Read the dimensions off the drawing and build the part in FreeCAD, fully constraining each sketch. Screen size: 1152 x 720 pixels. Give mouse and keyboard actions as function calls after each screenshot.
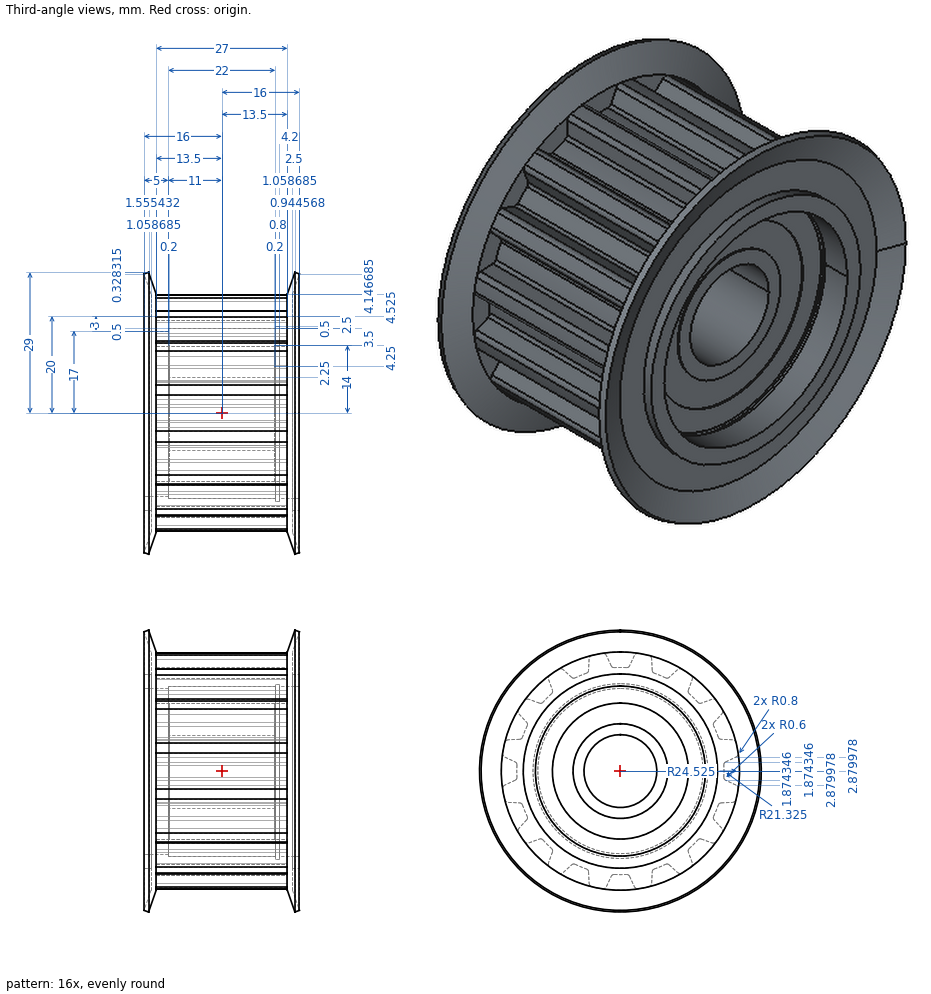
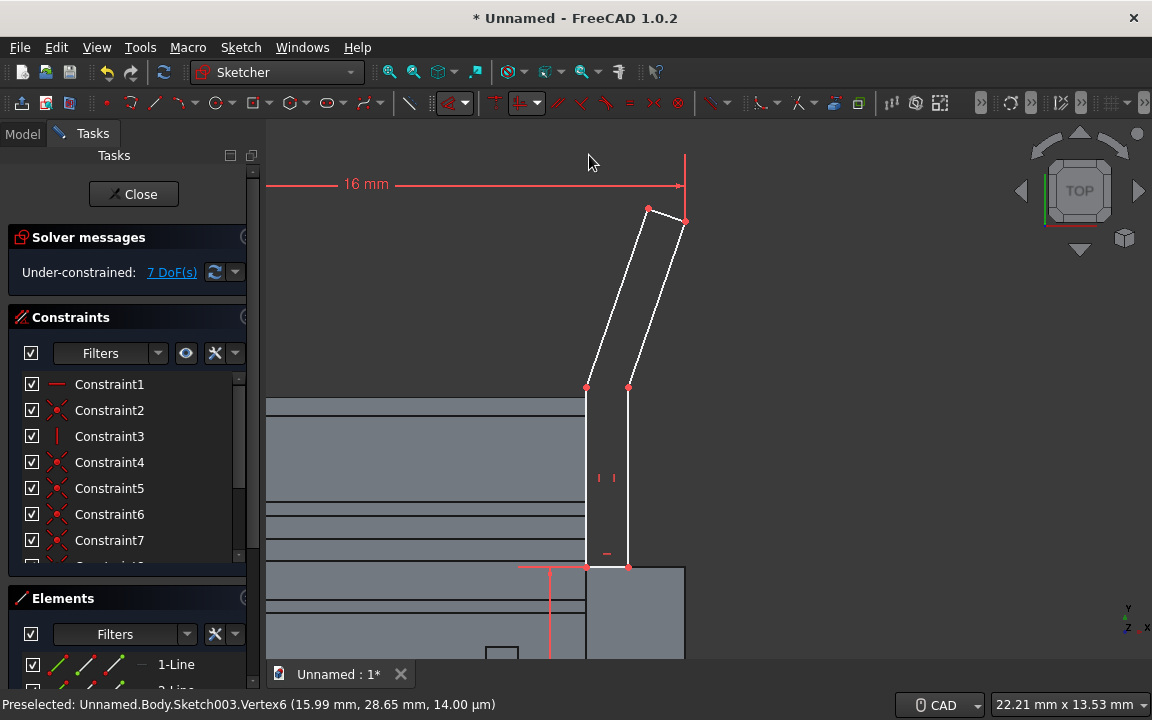
click(648, 209)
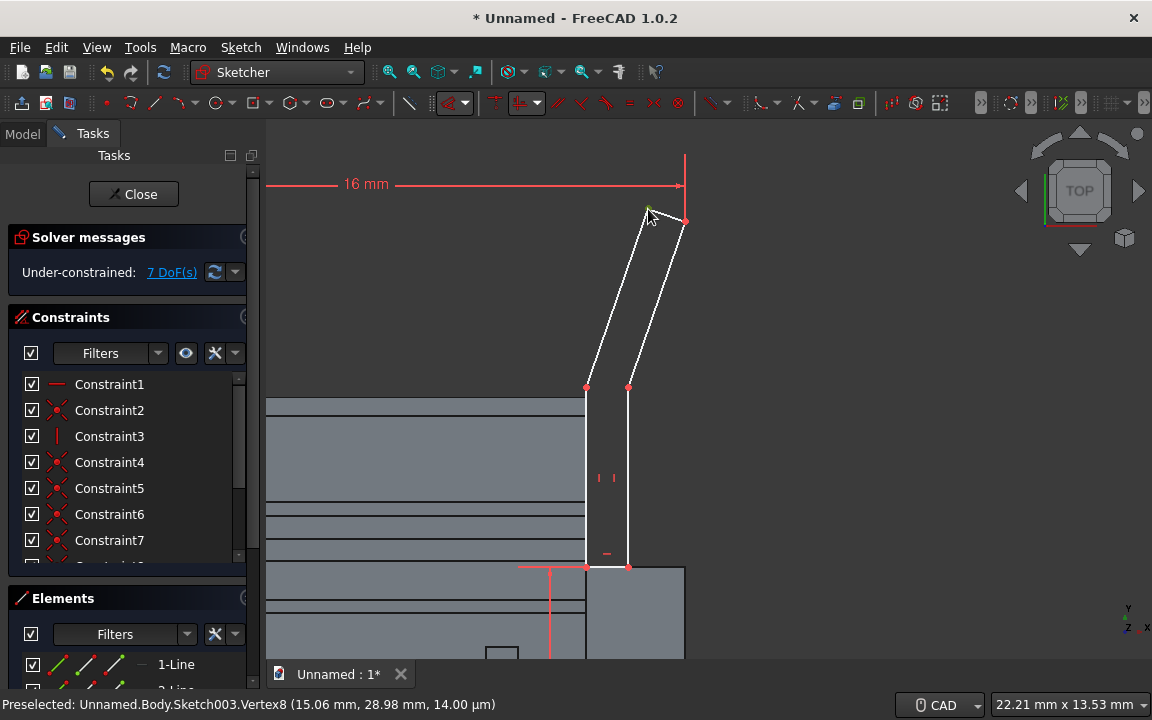
click(468, 104)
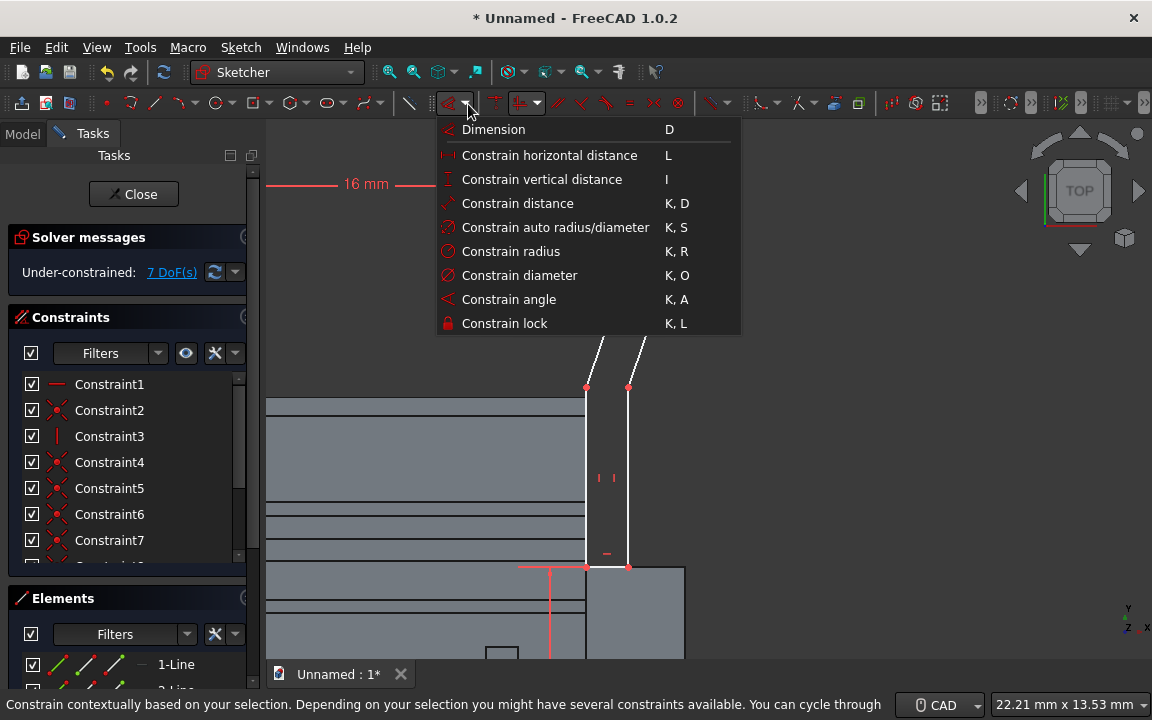
click(589, 179)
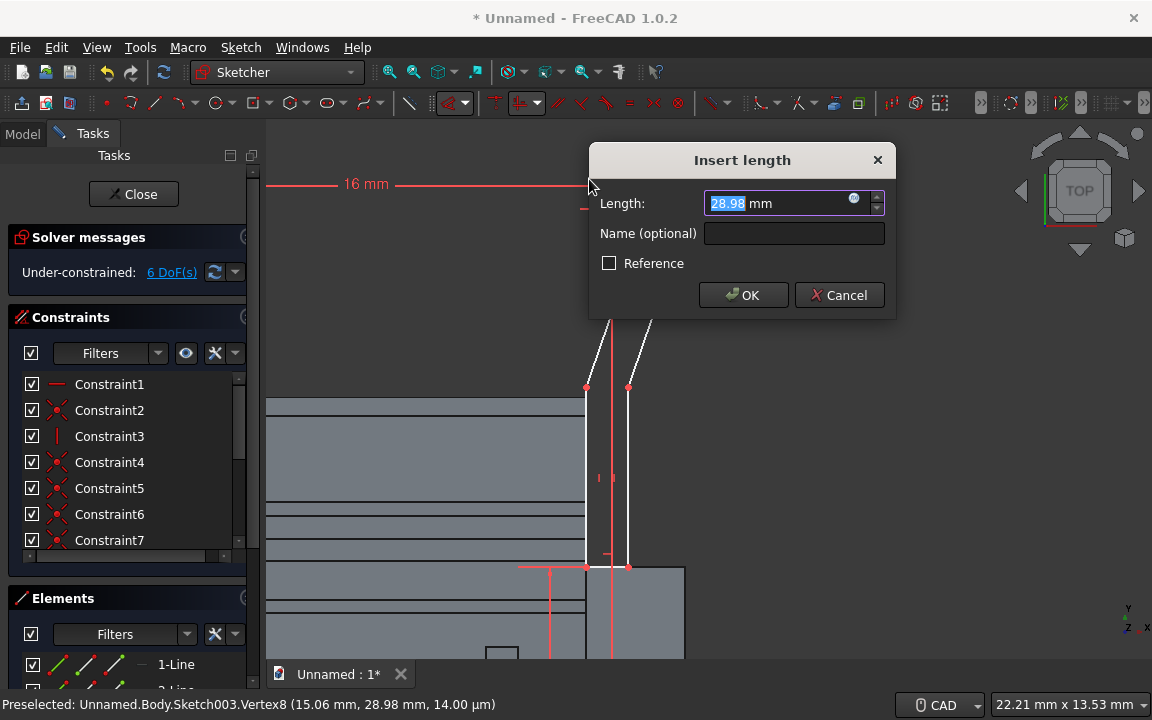
text(29)
key(Return)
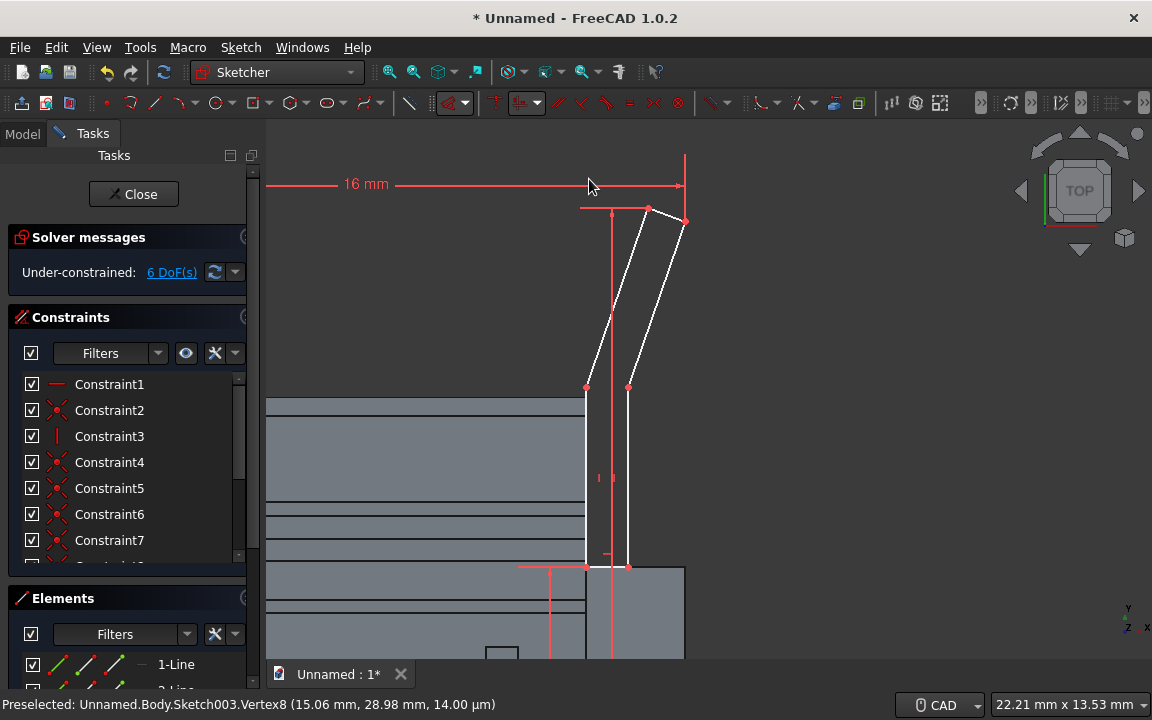
click(628, 513)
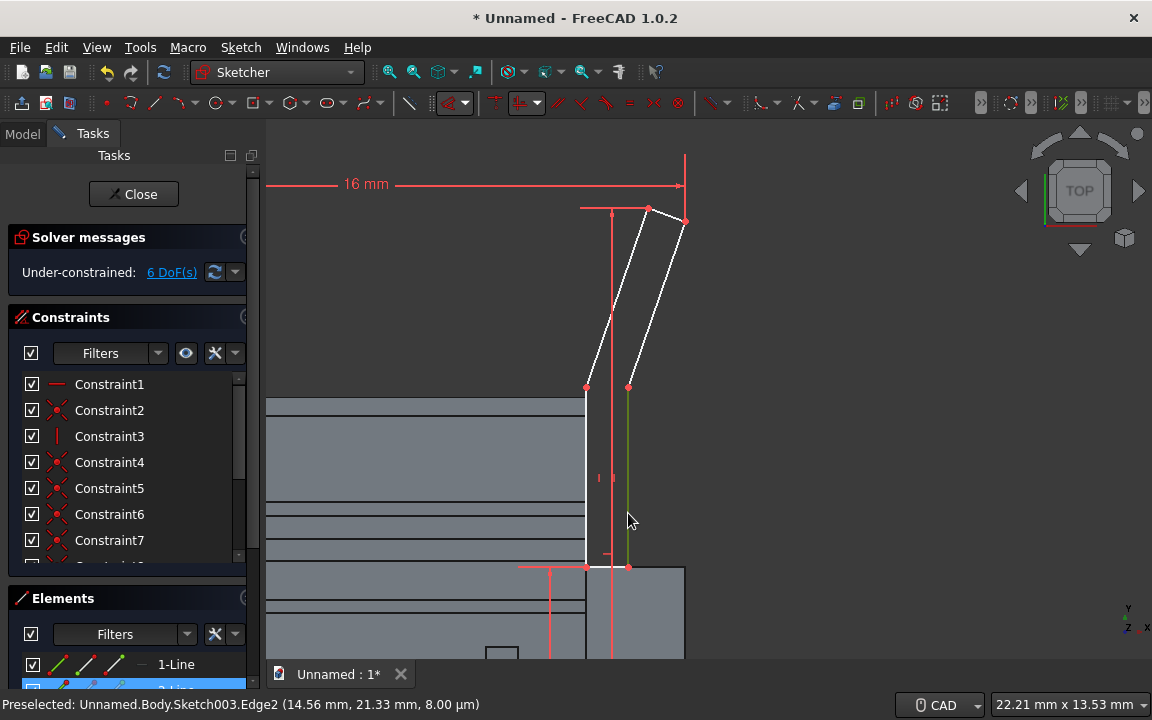
key(i)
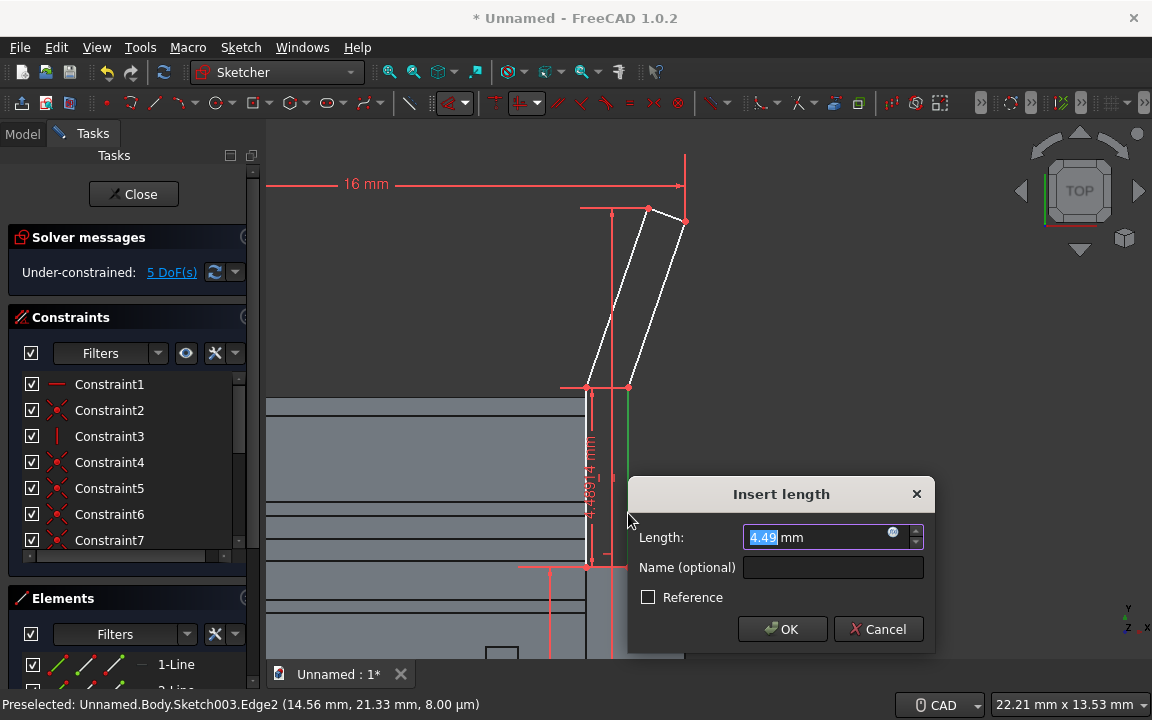
text(4.525)
key(Return)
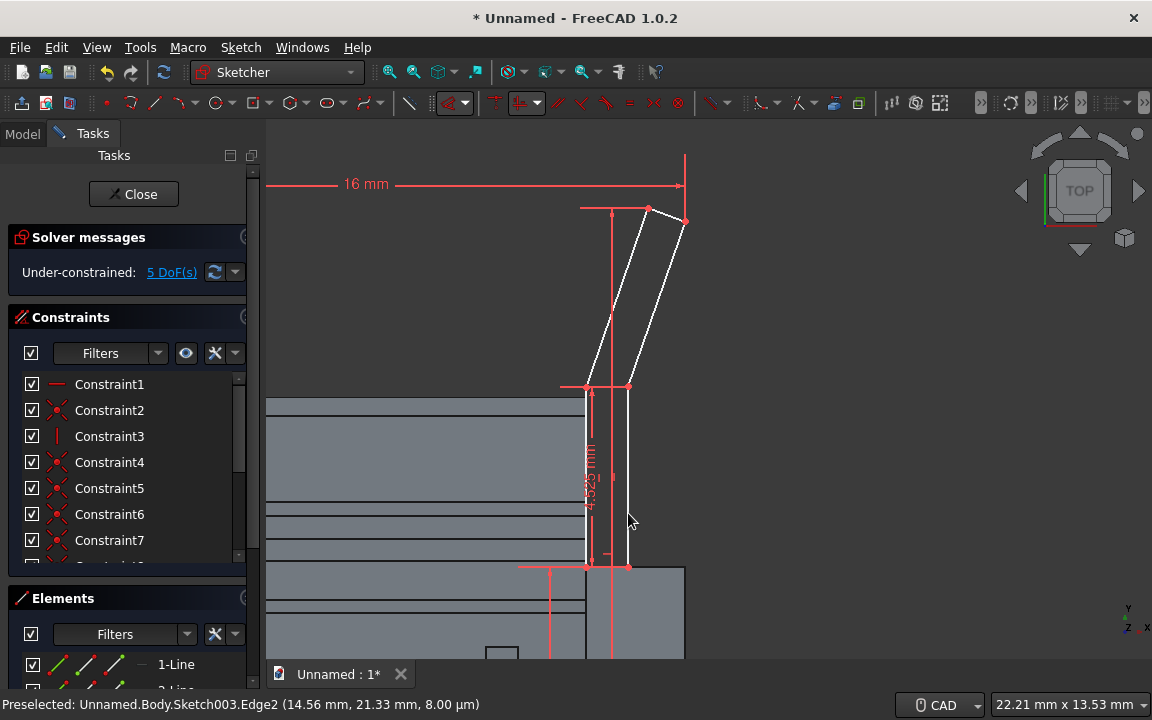
click(586, 442)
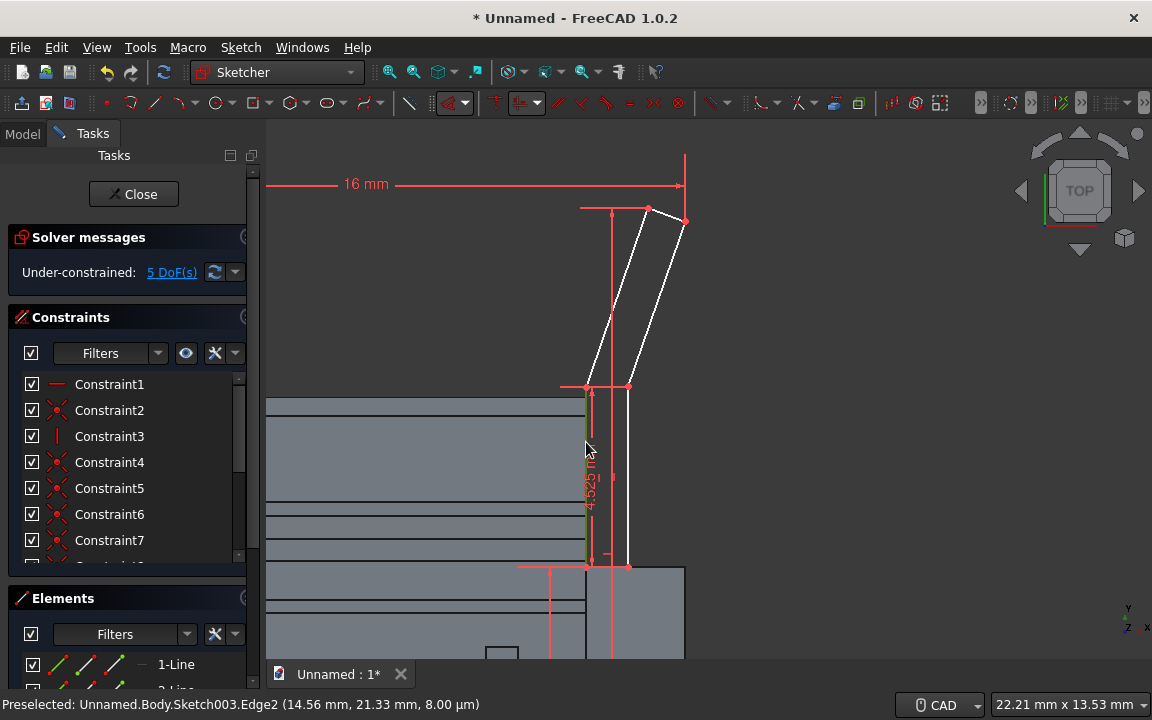
key(i)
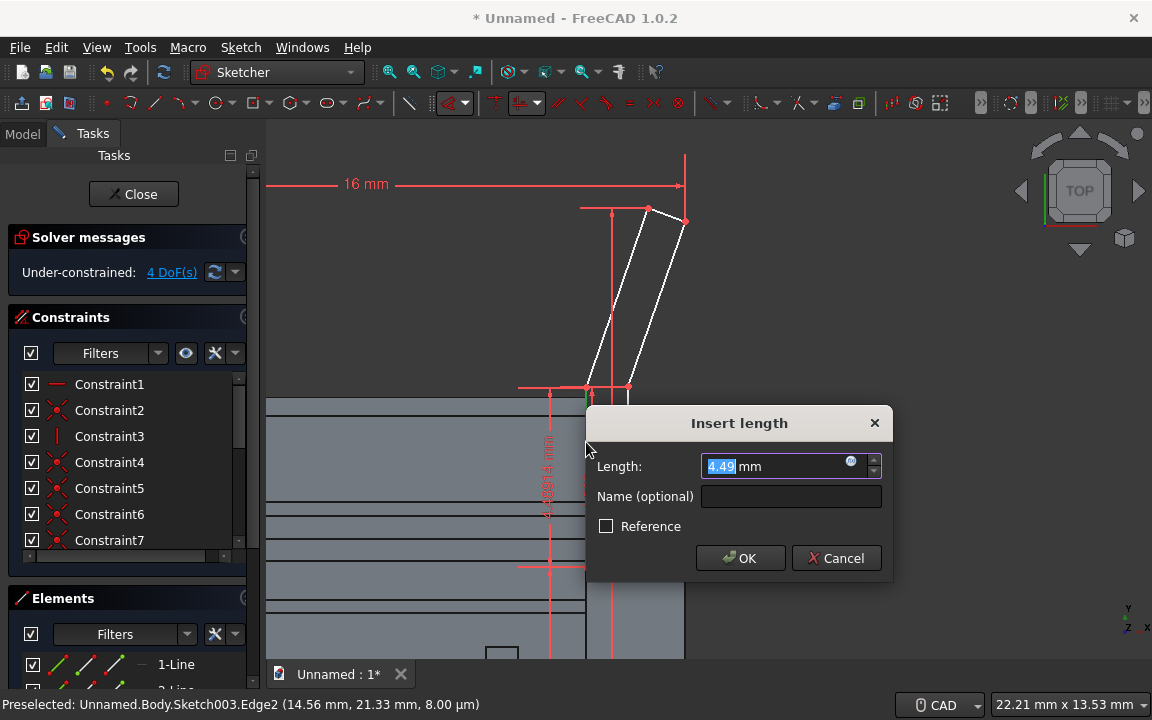
text(4.525)
key(Return)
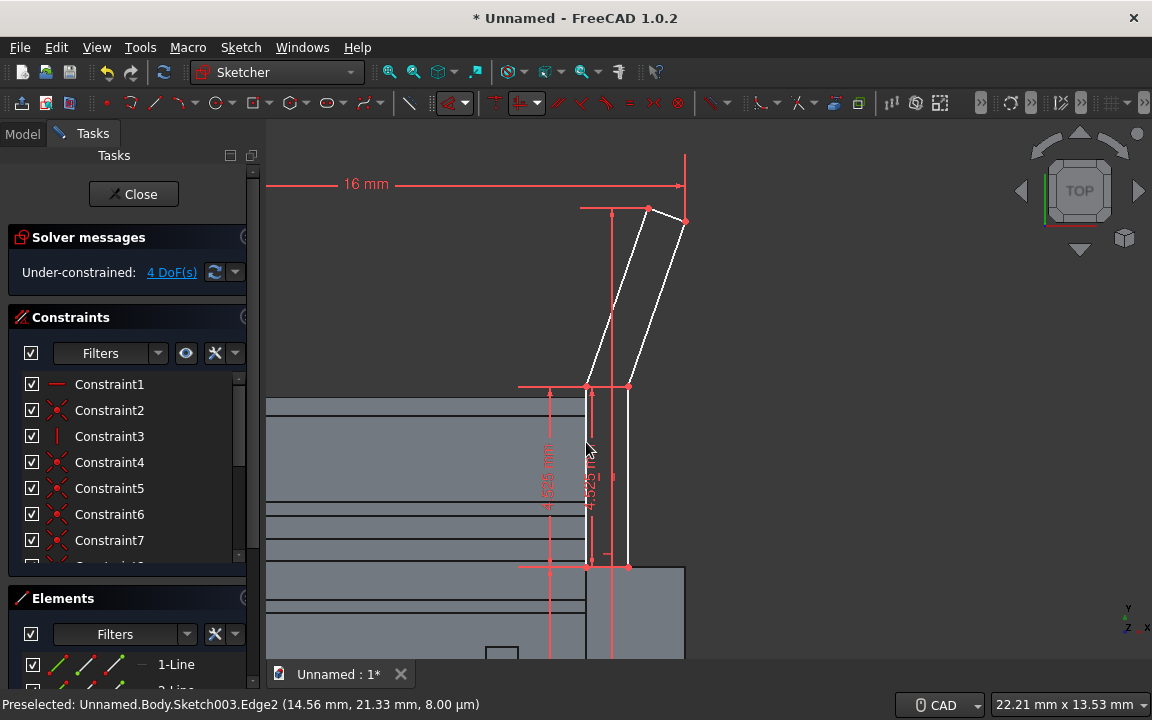
click(586, 567)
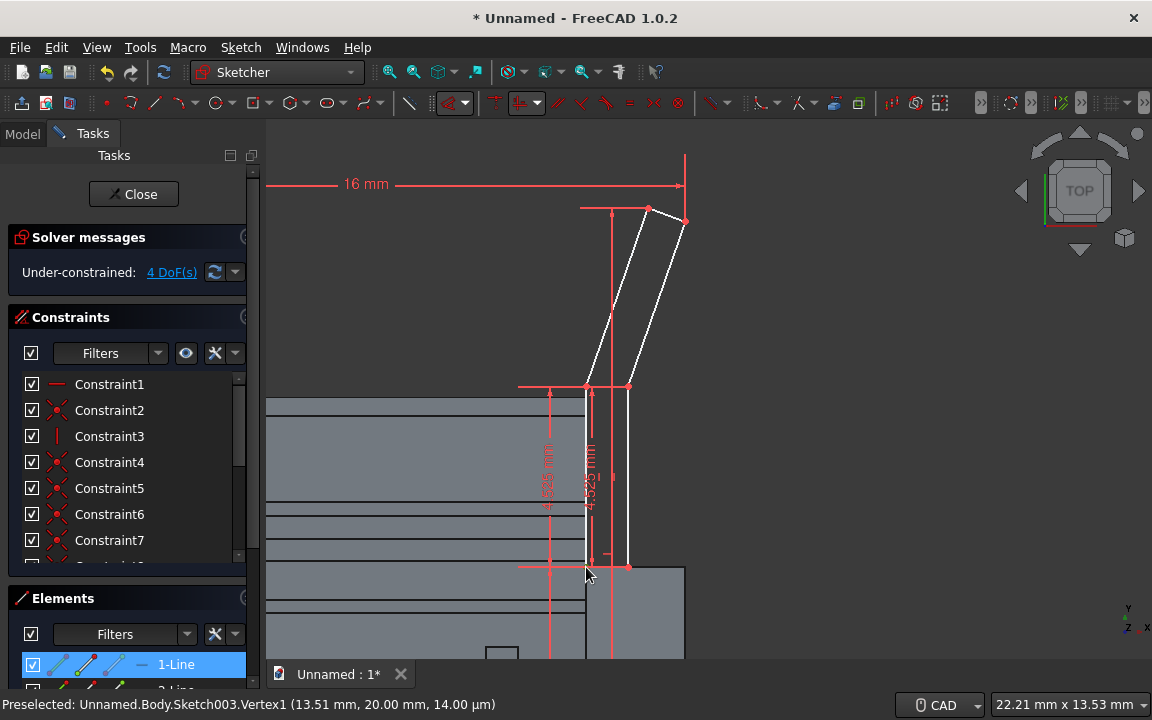
key(l)